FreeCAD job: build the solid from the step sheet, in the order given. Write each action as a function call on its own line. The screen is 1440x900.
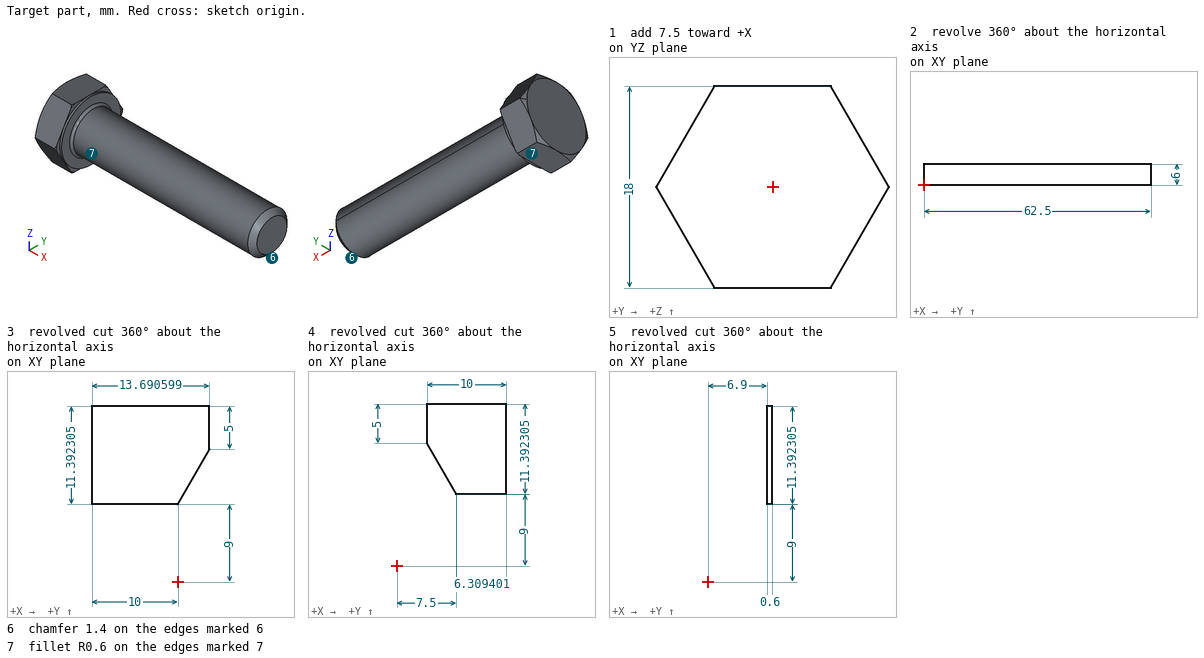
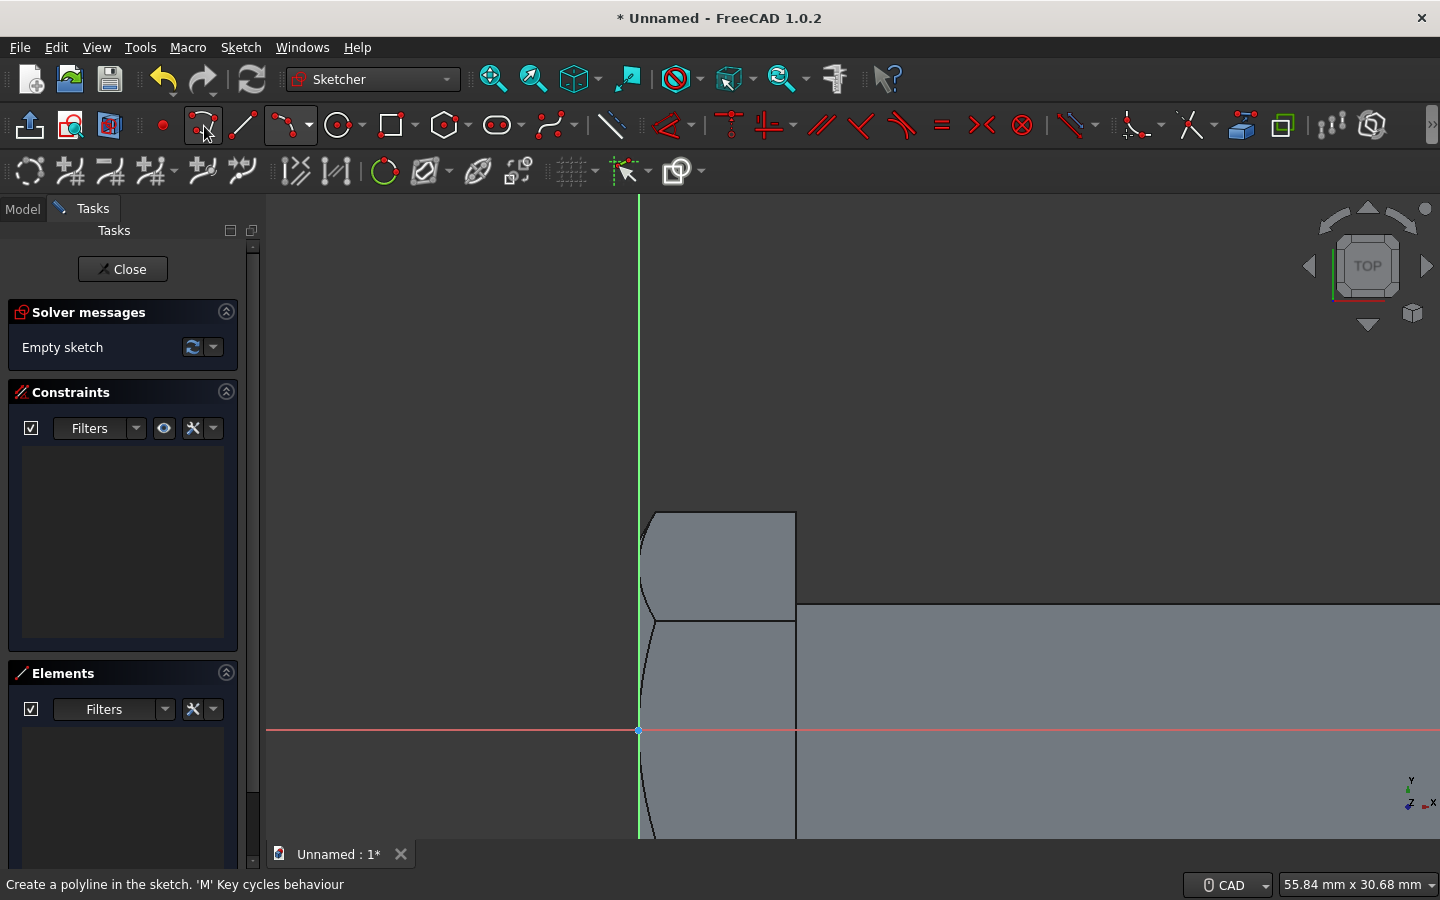
click(796, 541)
click(929, 541)
click(929, 302)
click(719, 302)
click(719, 407)
click(796, 542)
key(Escape)
key(Escape)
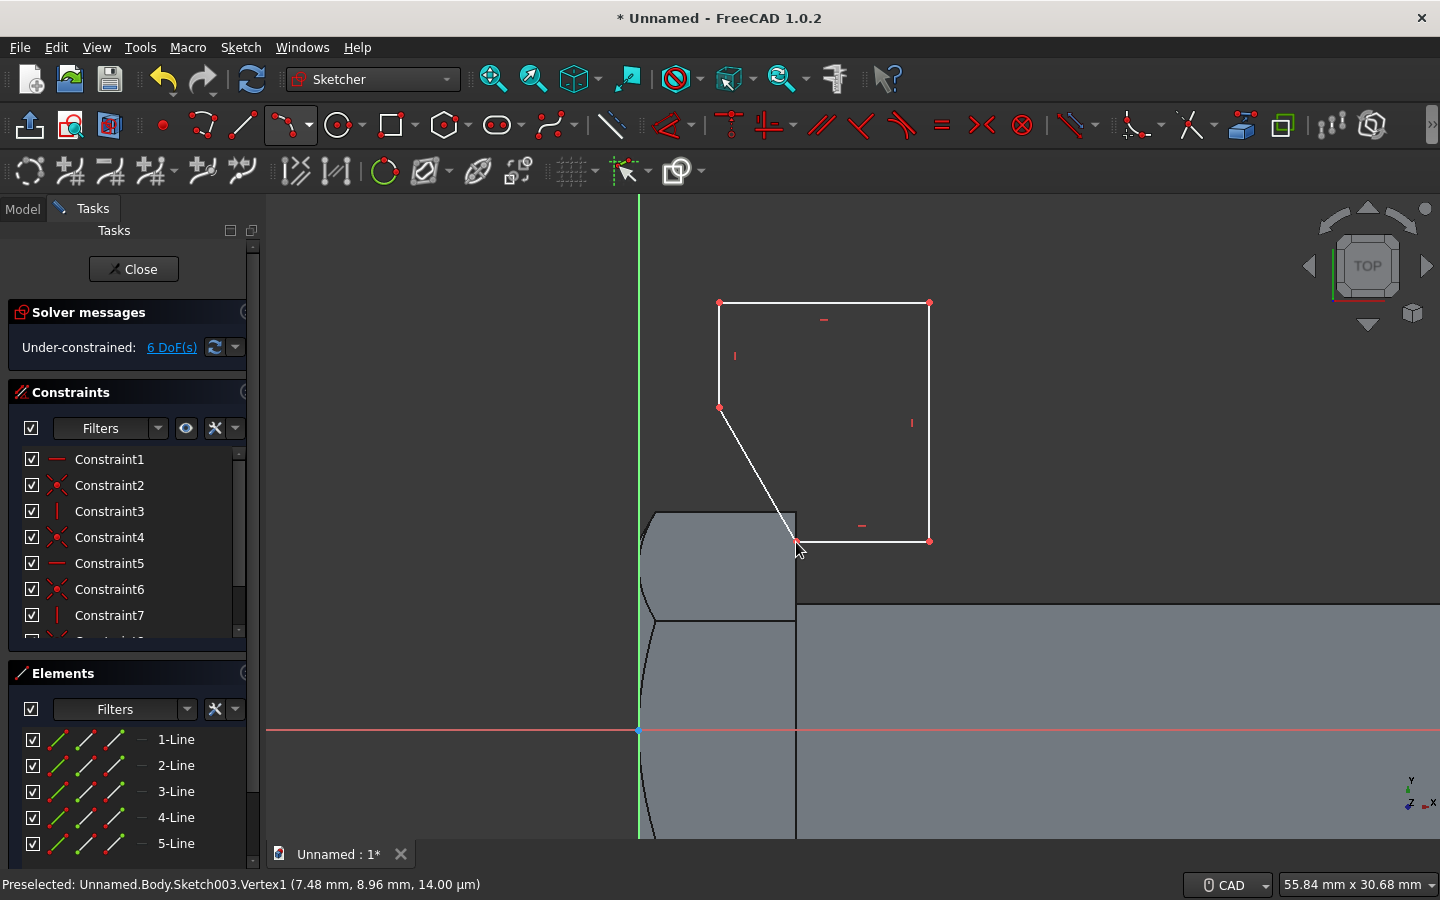
click(666, 126)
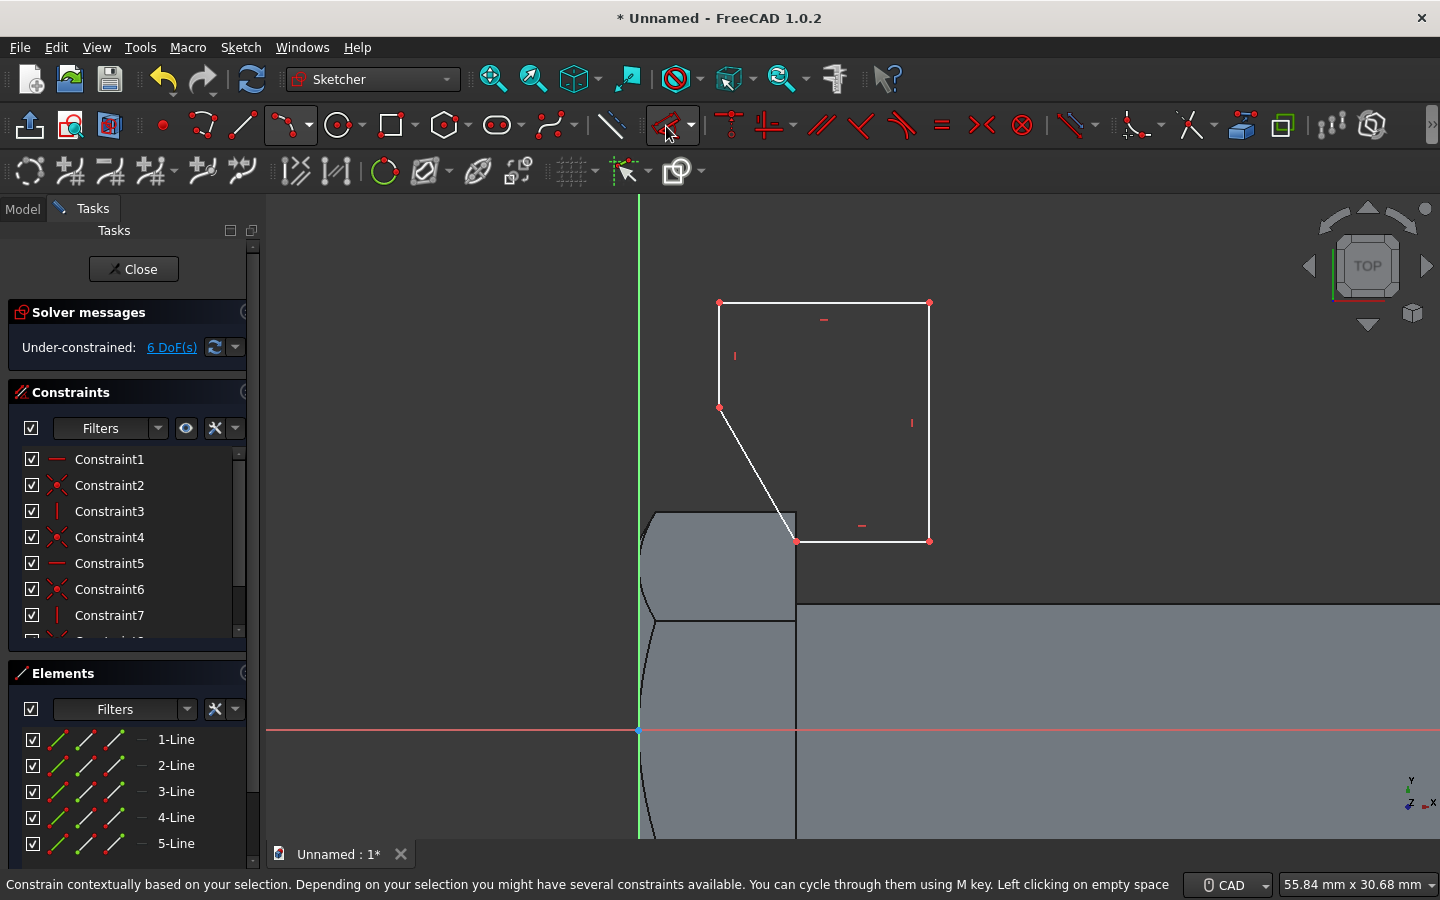
click(719, 334)
click(685, 355)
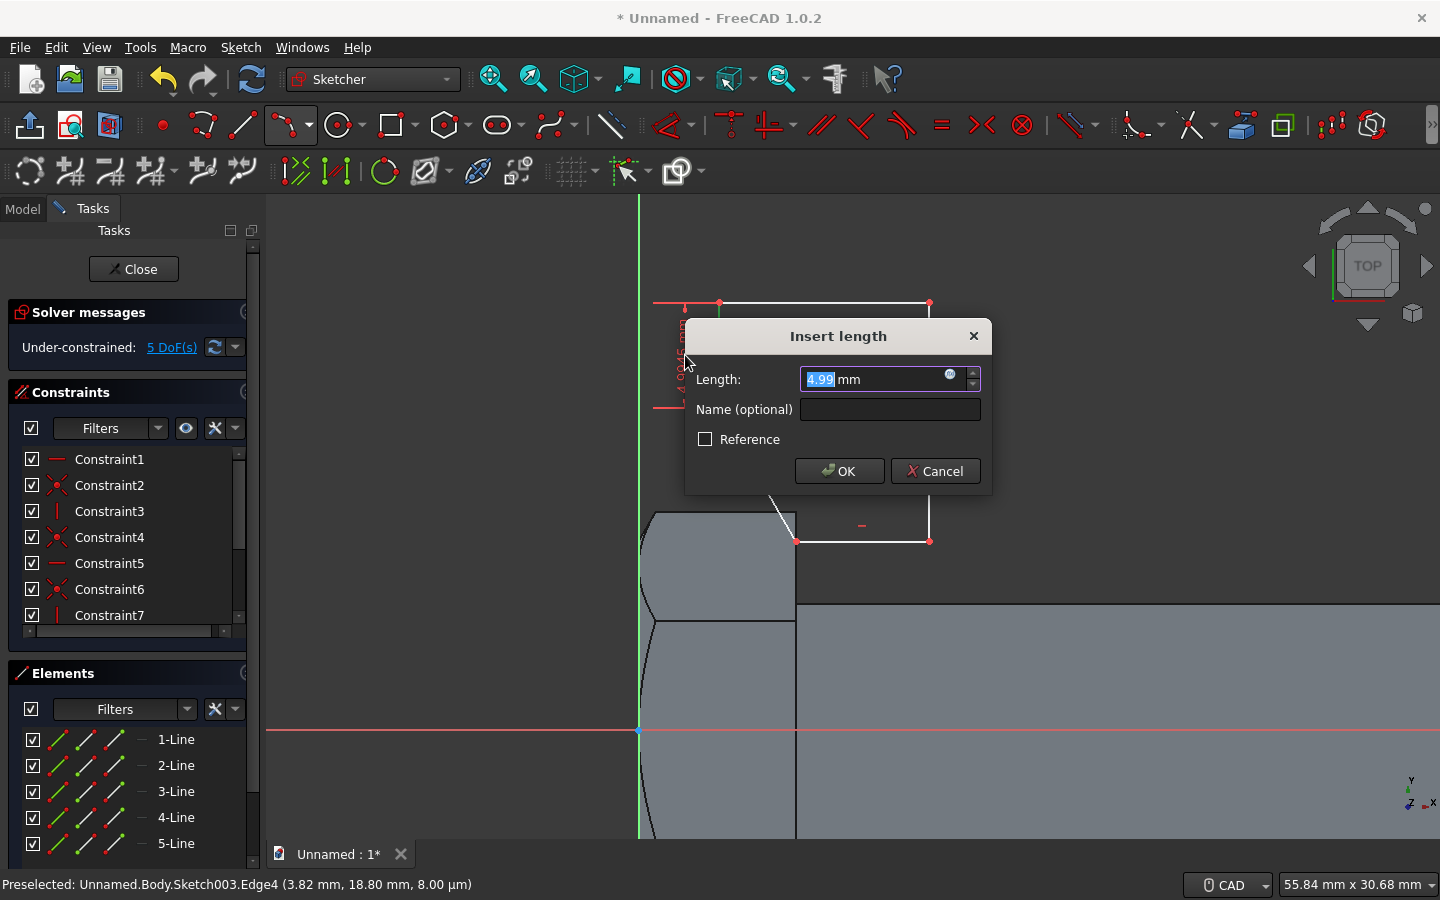
text(5)
key(Return)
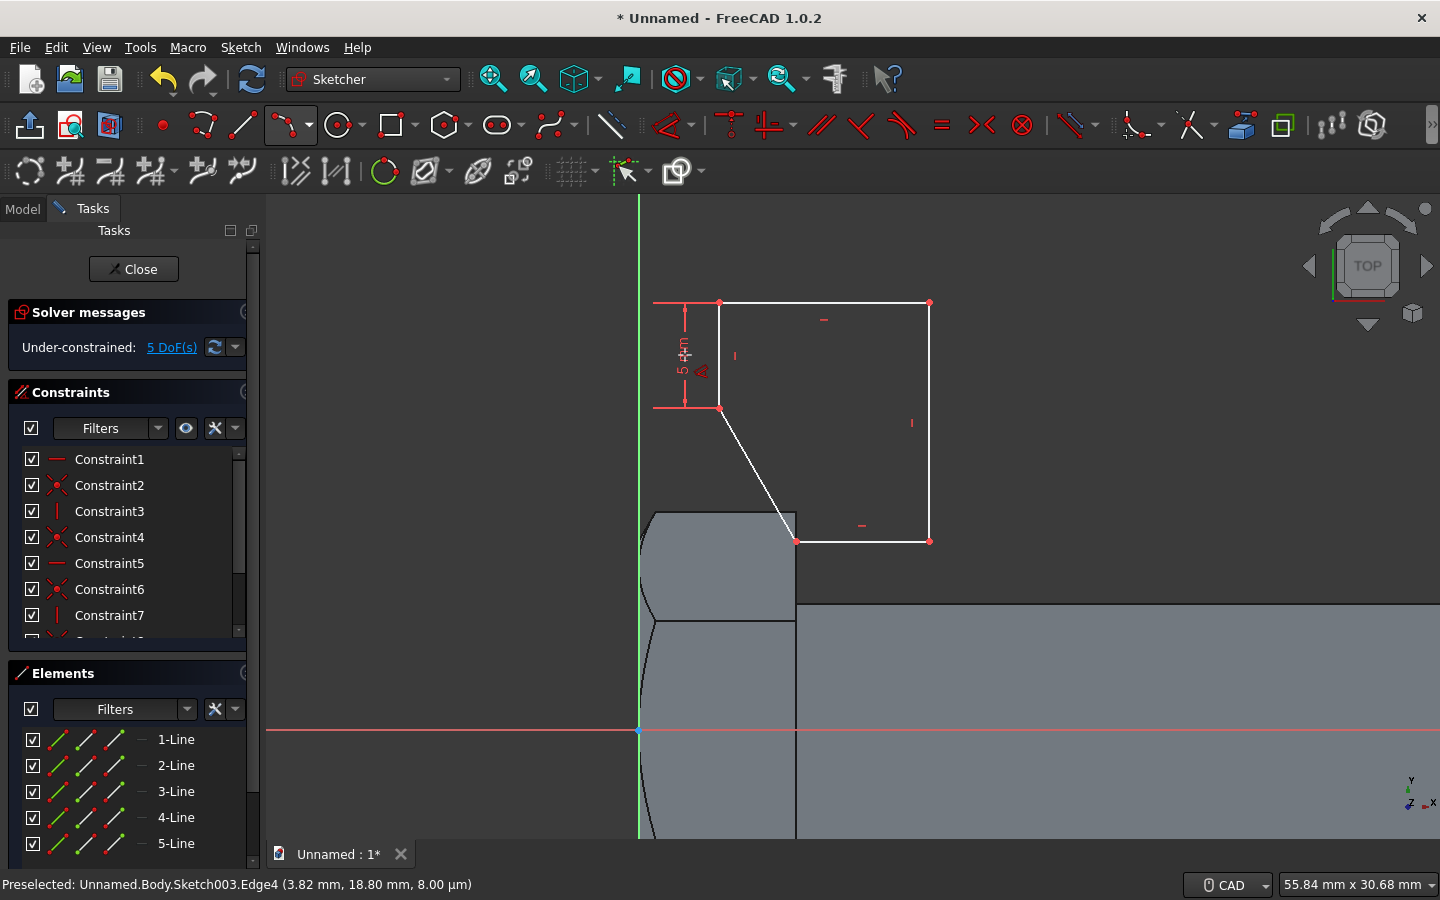
click(866, 303)
click(824, 269)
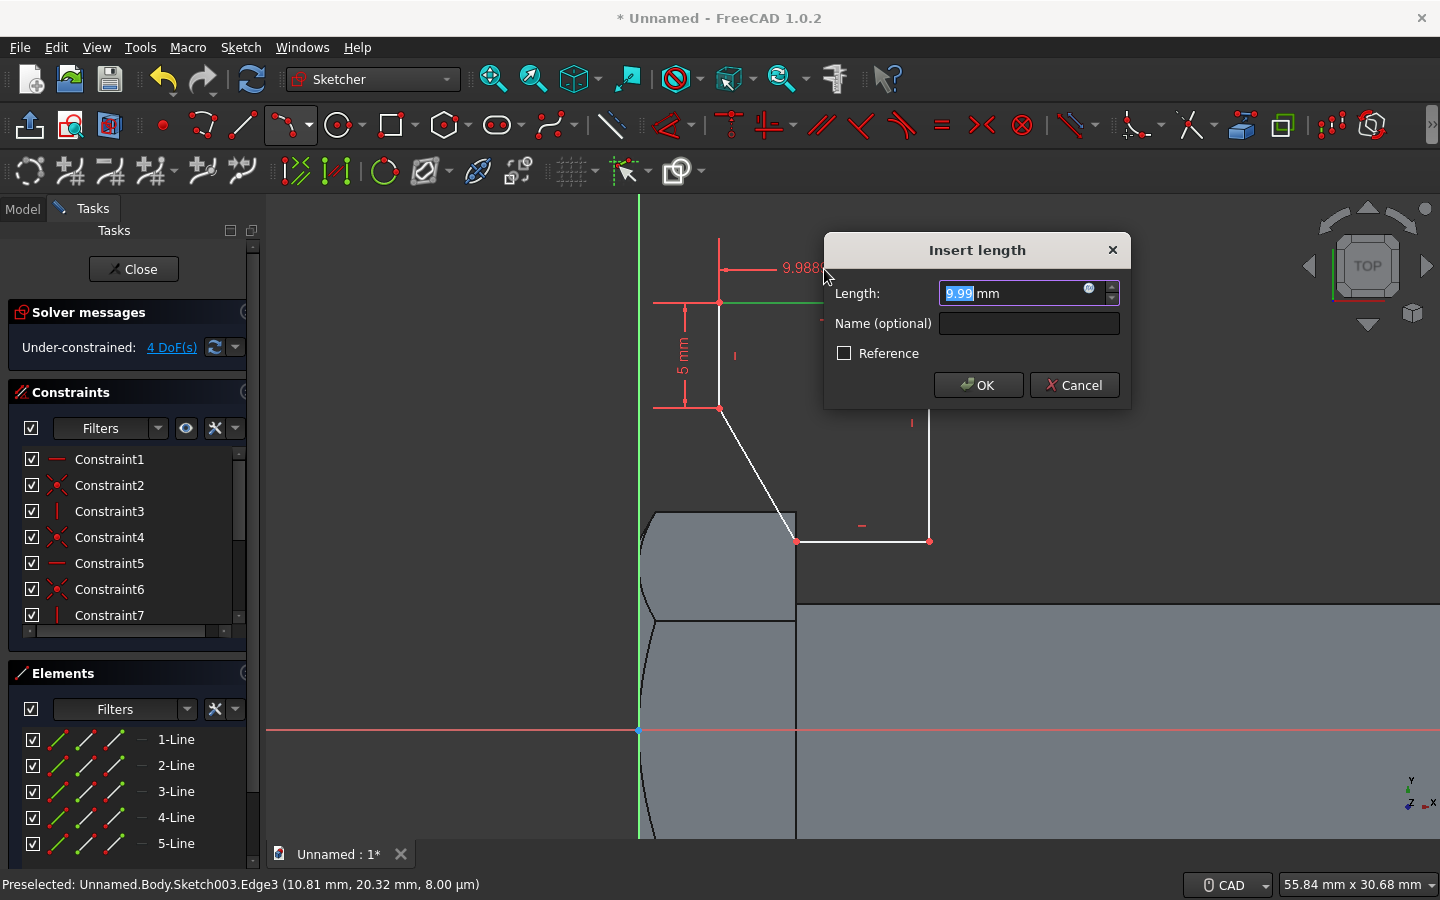
text(10)
key(Return)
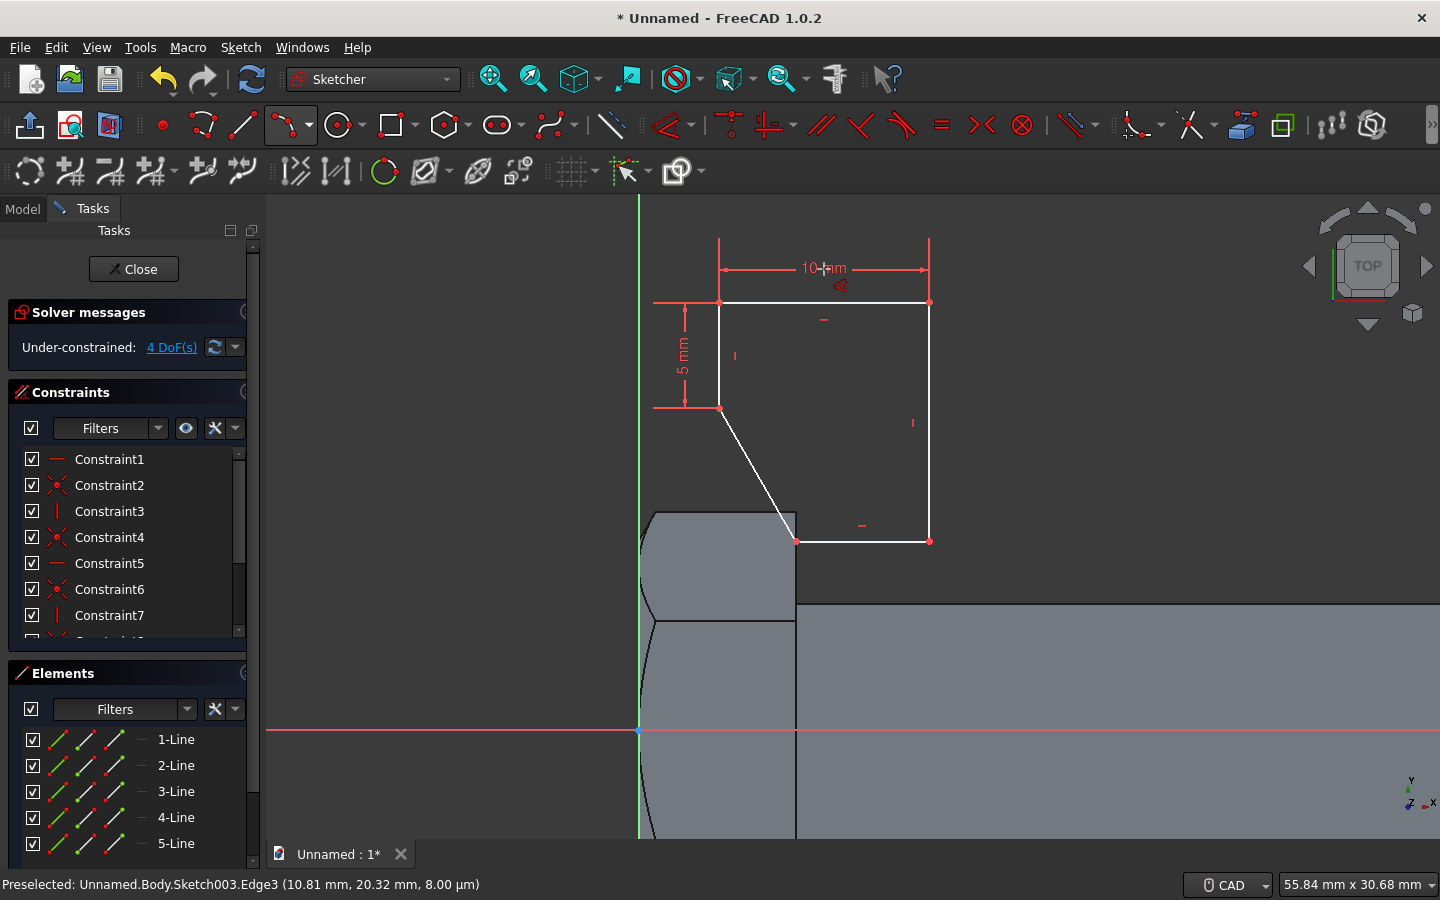
click(796, 542)
click(605, 636)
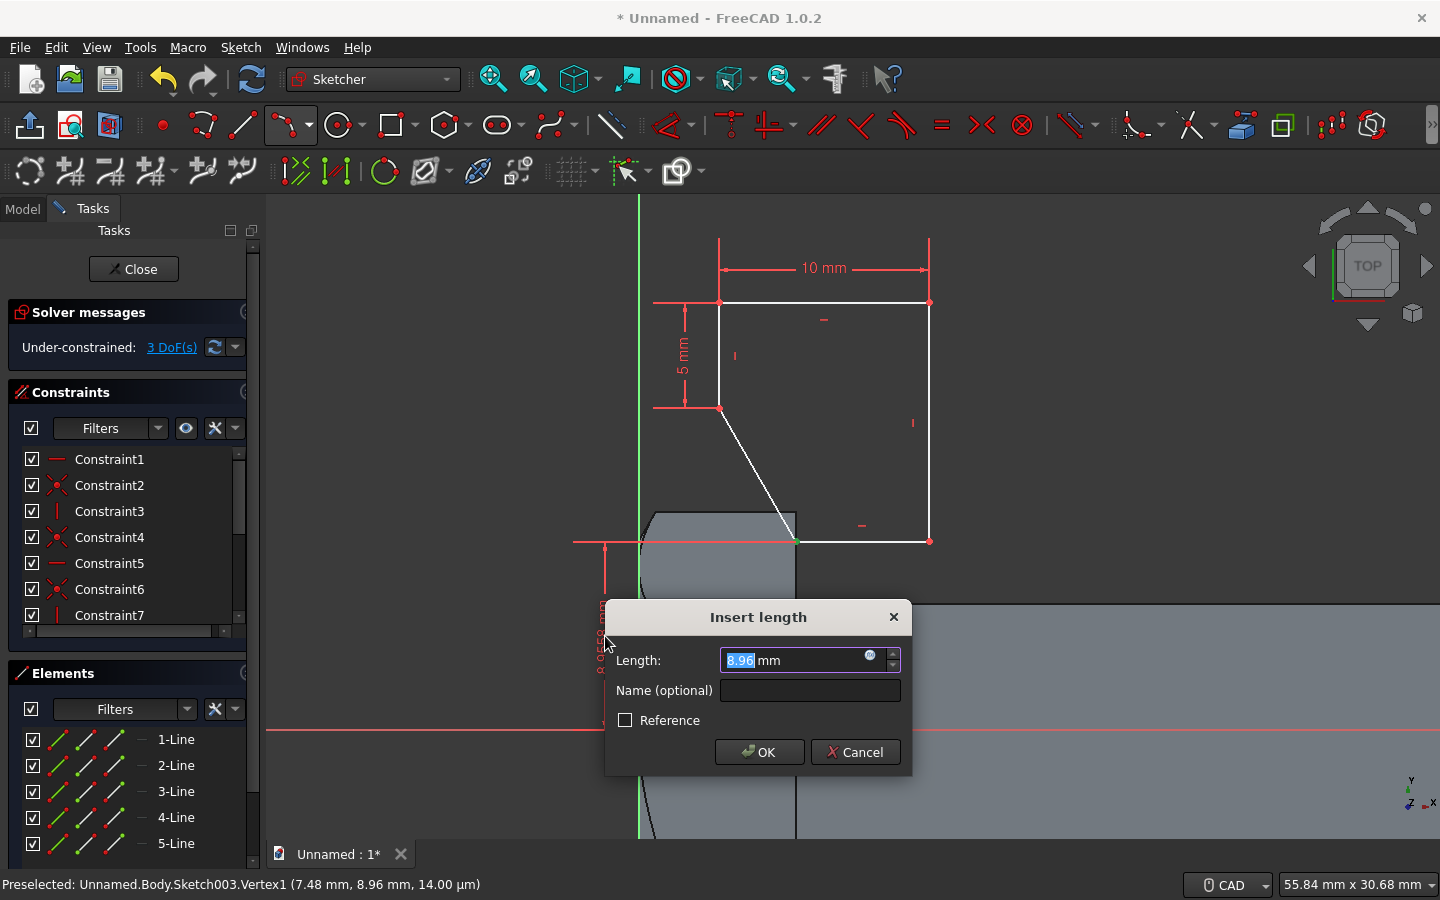
text(9)
key(Return)